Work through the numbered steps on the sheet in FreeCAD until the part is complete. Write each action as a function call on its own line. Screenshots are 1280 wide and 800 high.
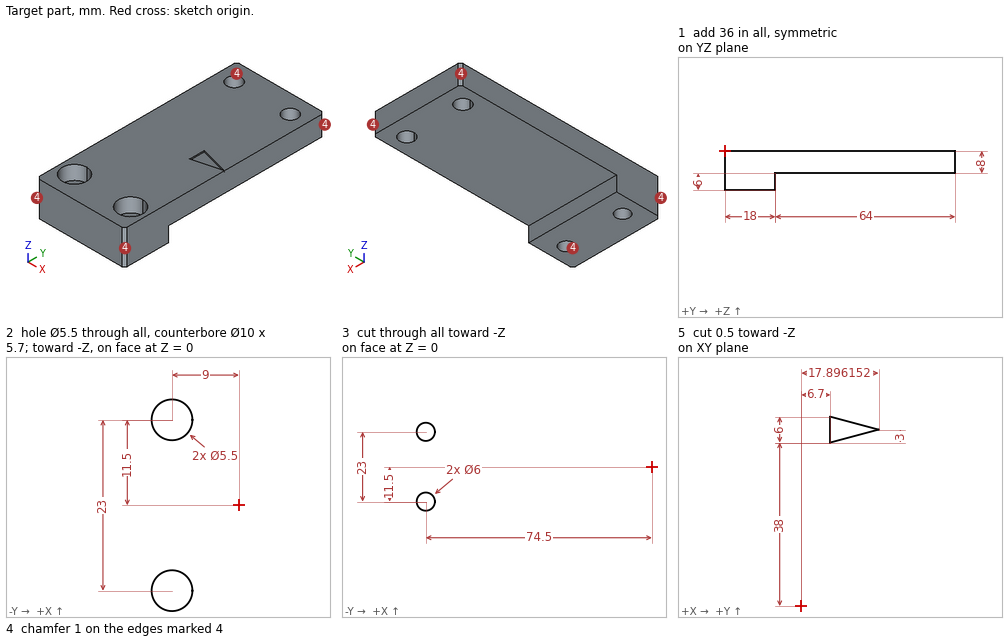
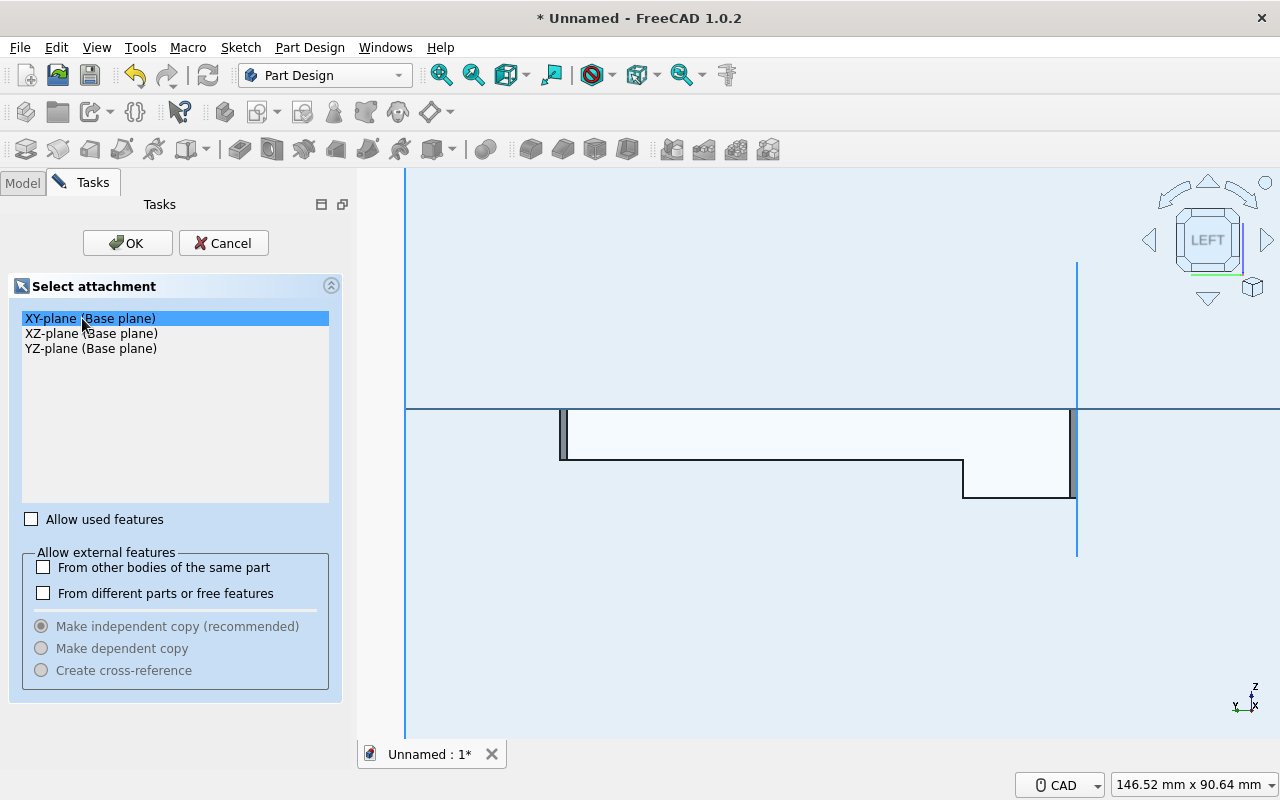
click(128, 243)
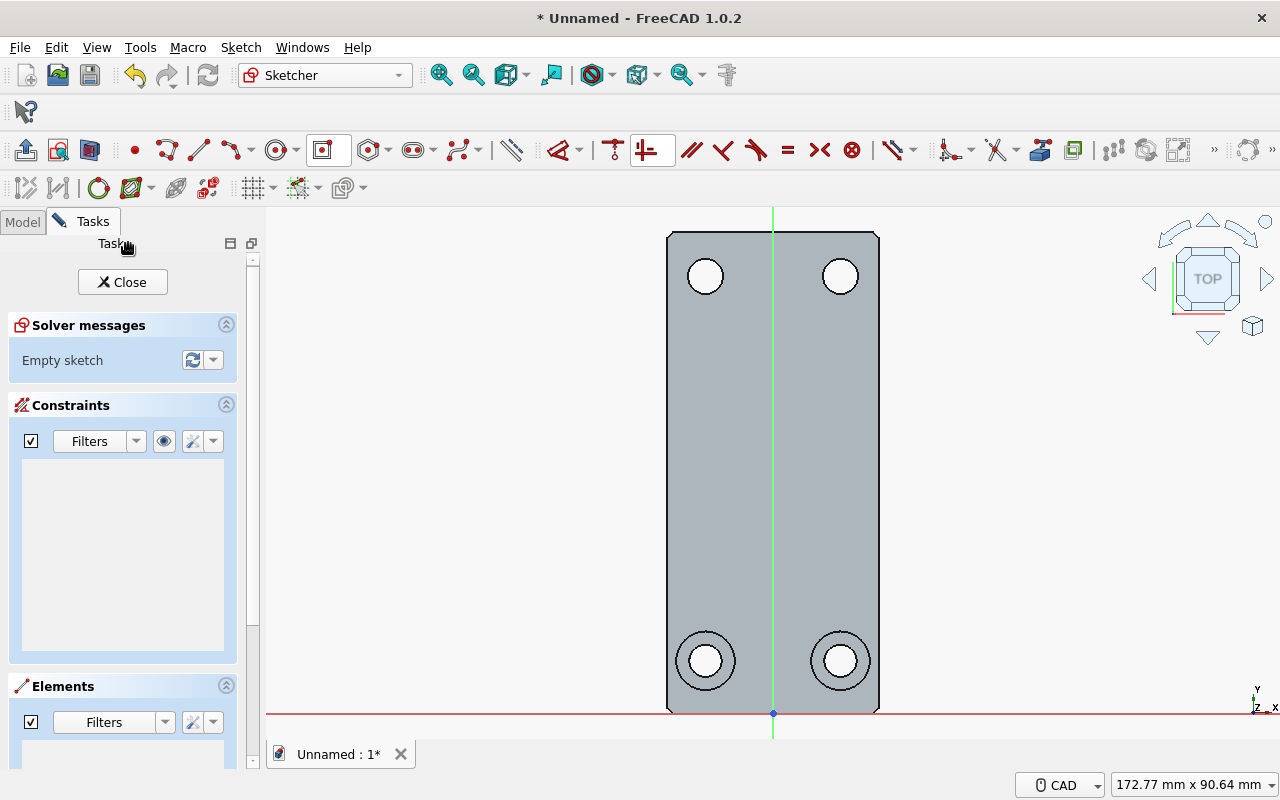
scroll(863, 473, up, 11)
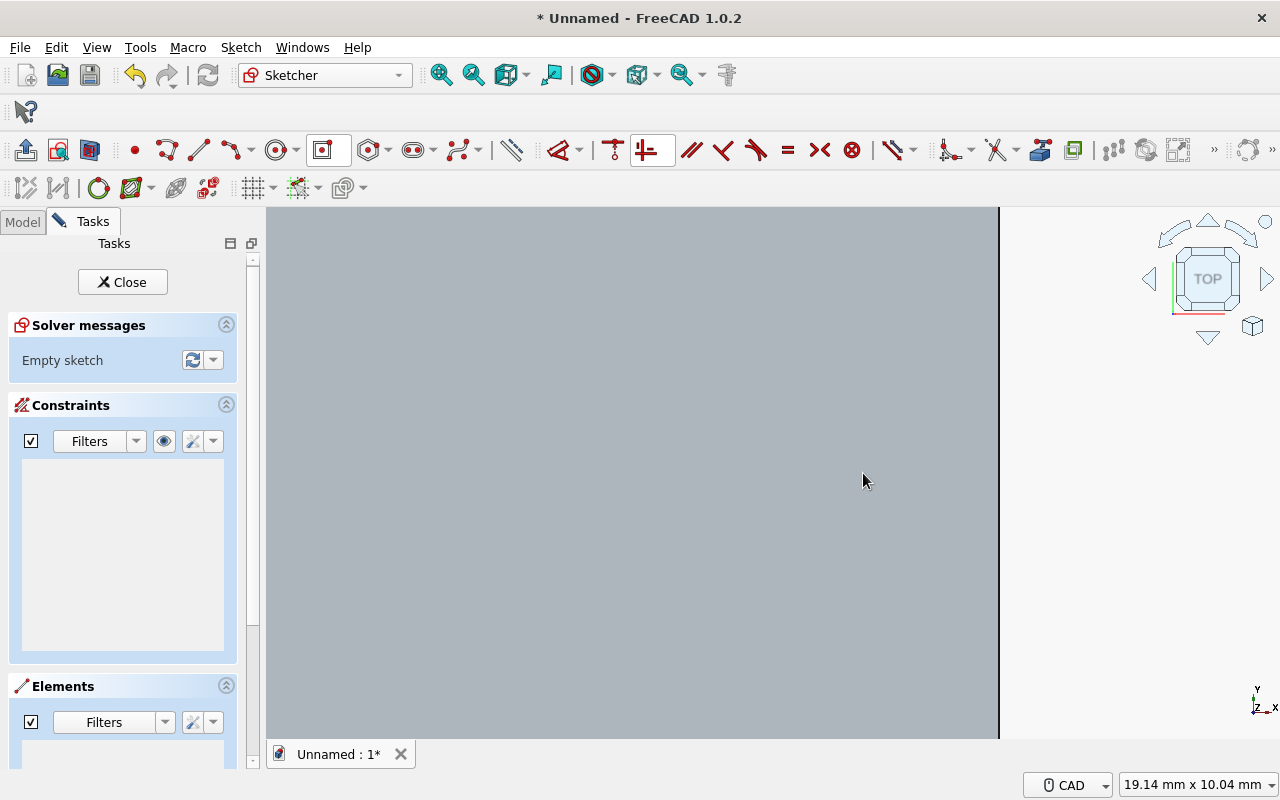
key(g)
key(m)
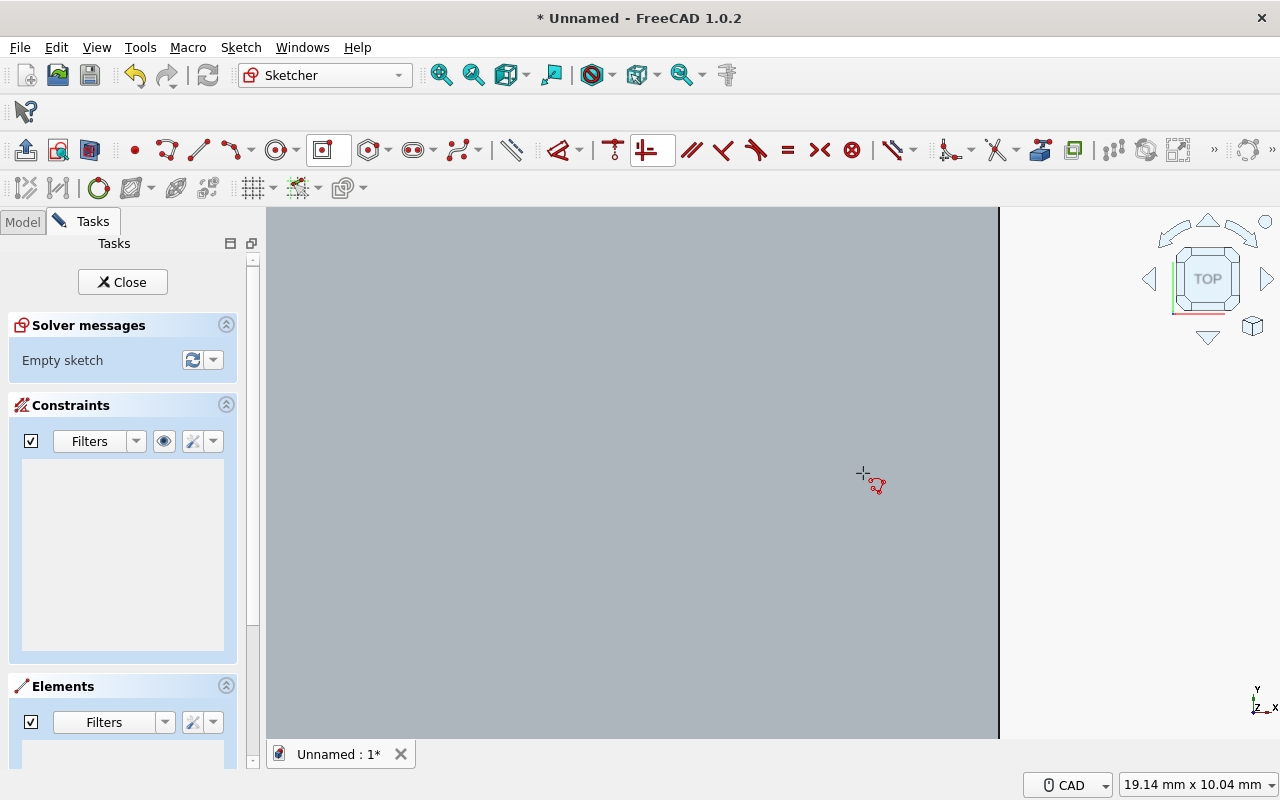
click(401, 628)
click(994, 469)
click(401, 310)
click(401, 629)
key(Escape)
key(Escape)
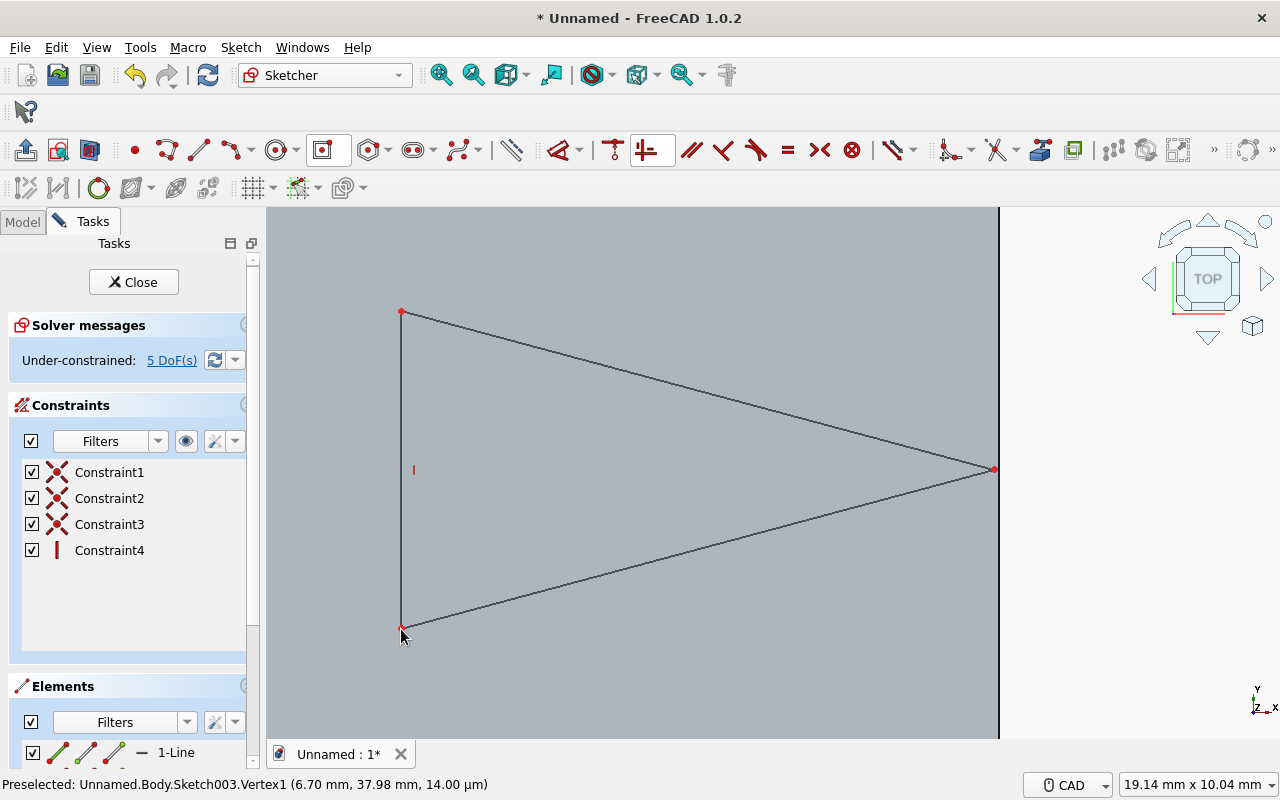
click(558, 150)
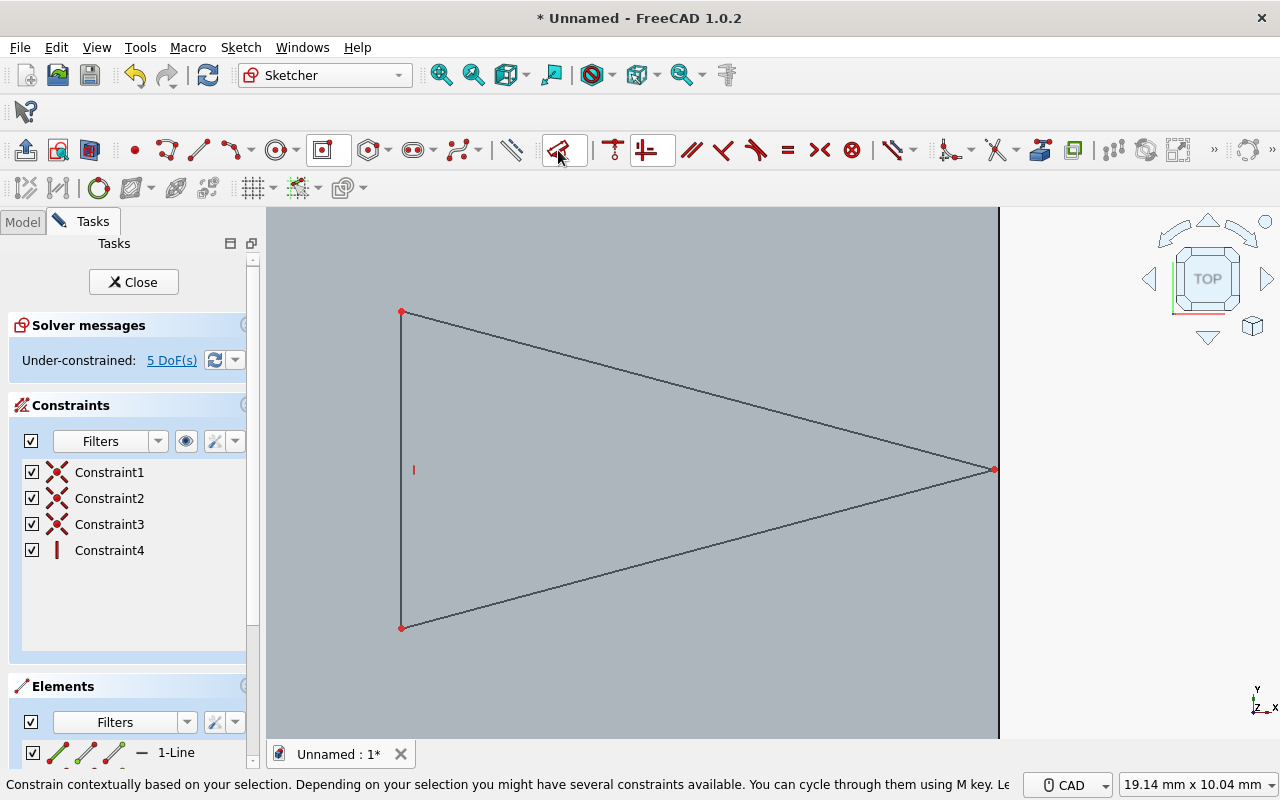
click(401, 406)
click(367, 470)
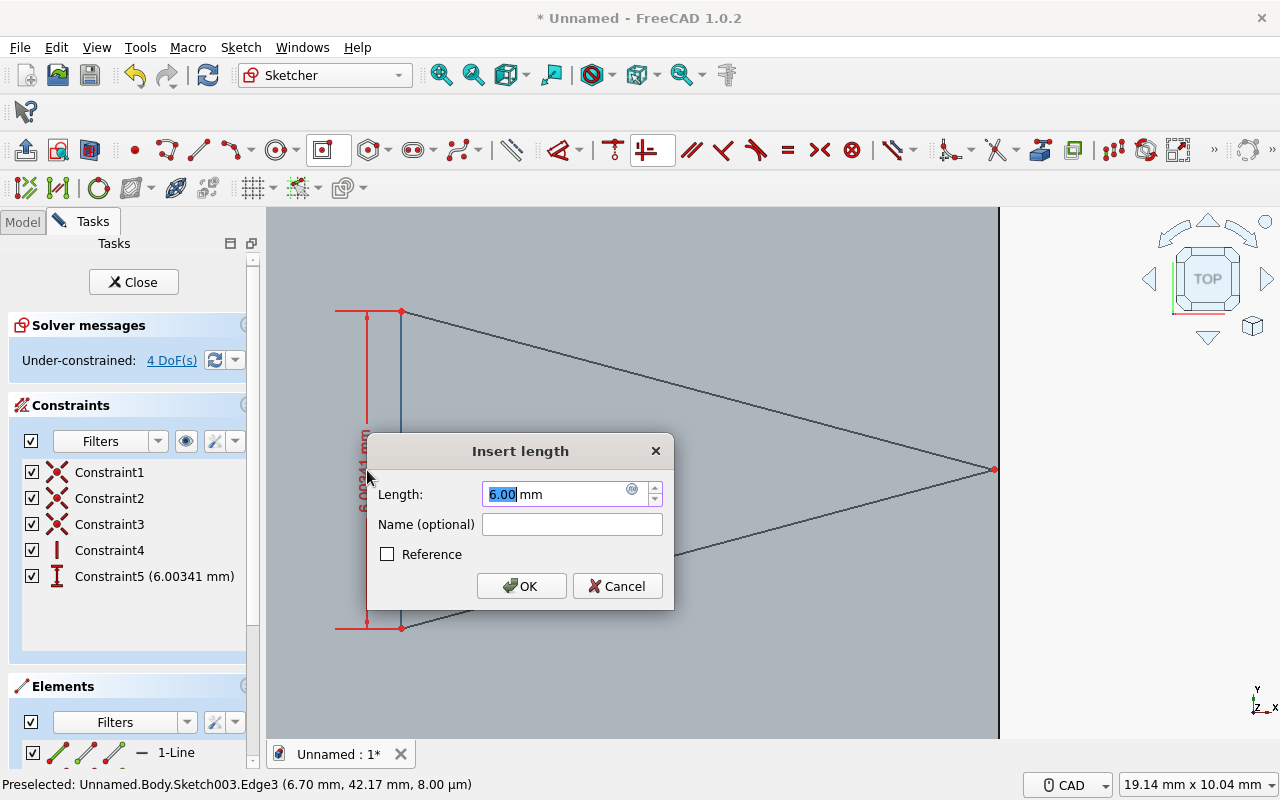
text(6)
key(Return)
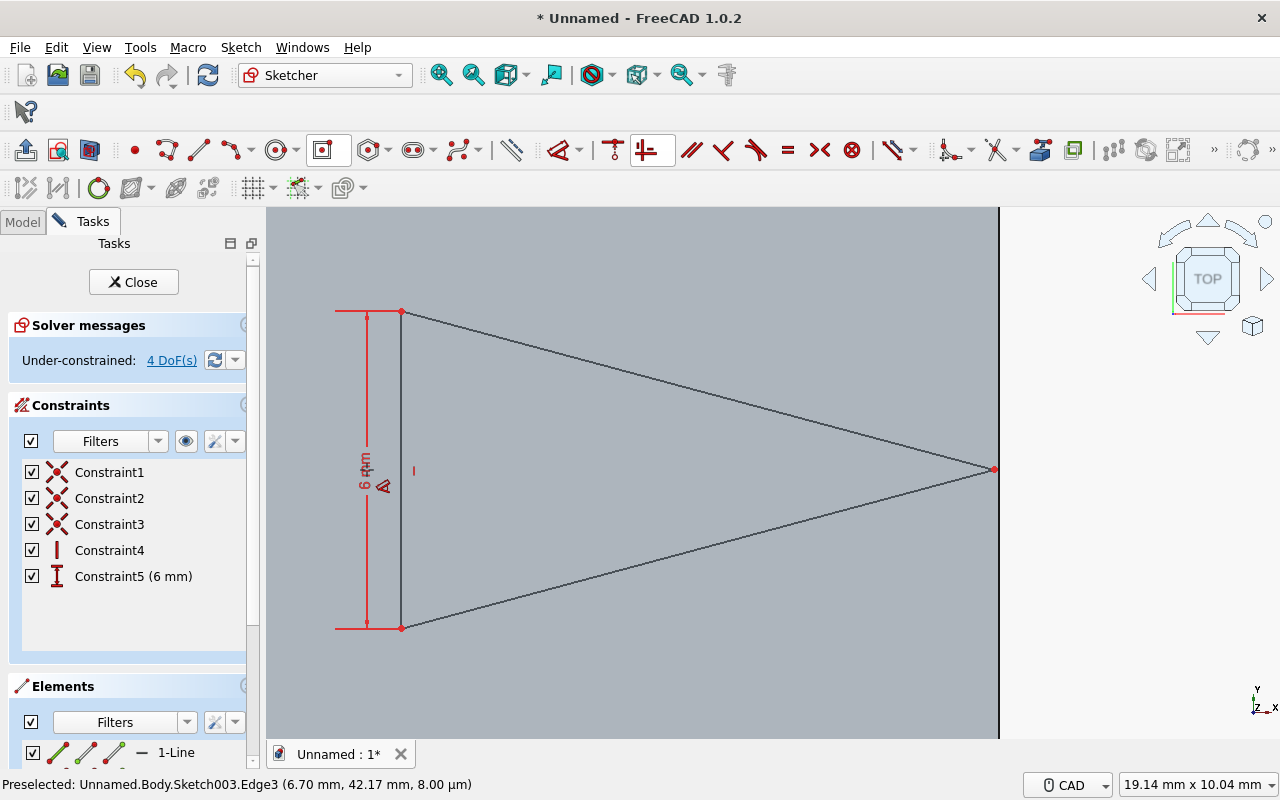
click(579, 581)
click(1028, 549)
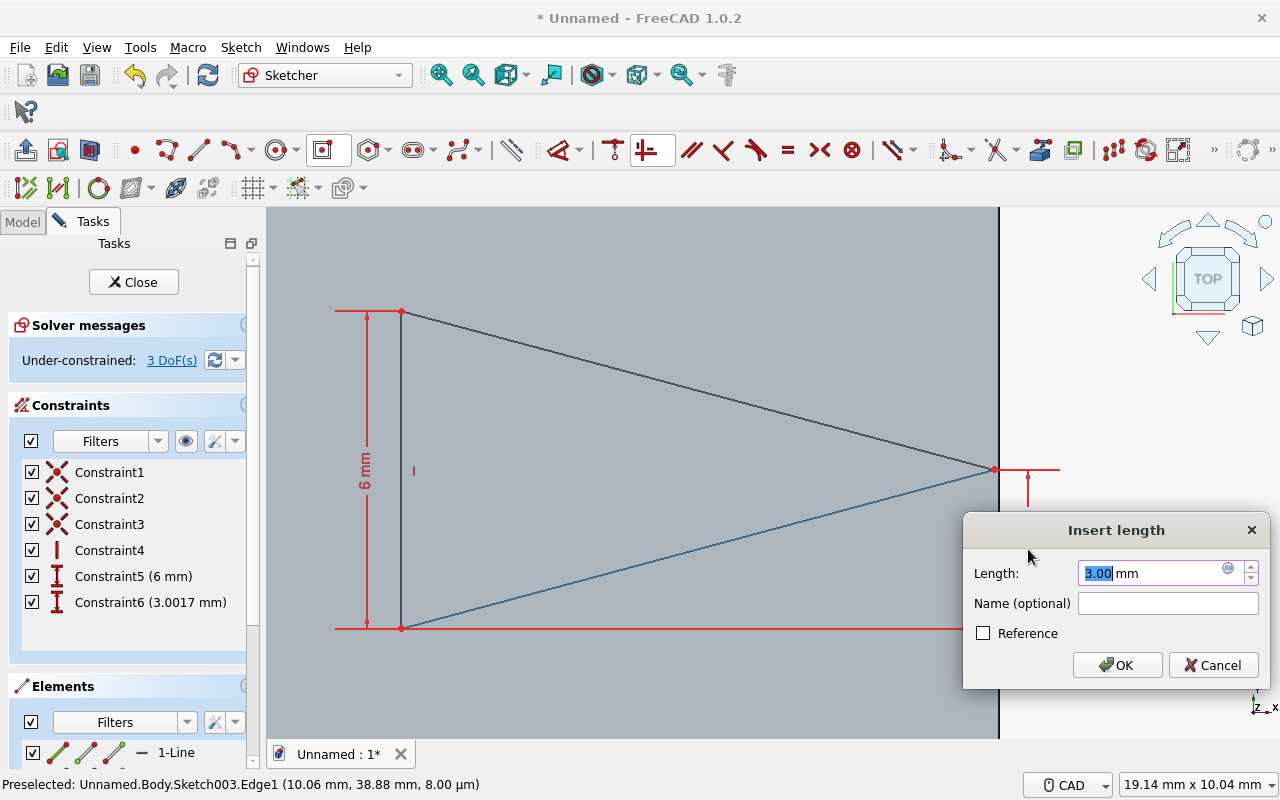
text(3)
key(Return)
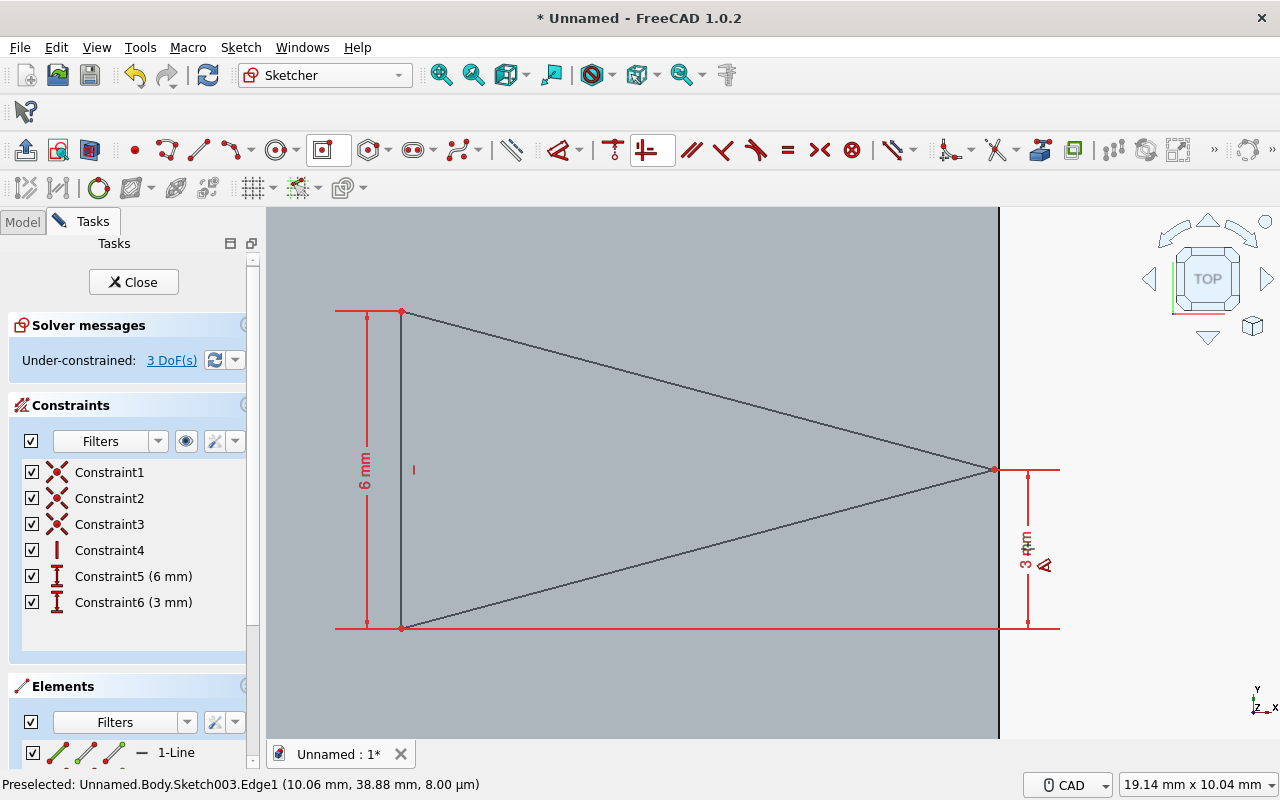
click(401, 629)
click(435, 670)